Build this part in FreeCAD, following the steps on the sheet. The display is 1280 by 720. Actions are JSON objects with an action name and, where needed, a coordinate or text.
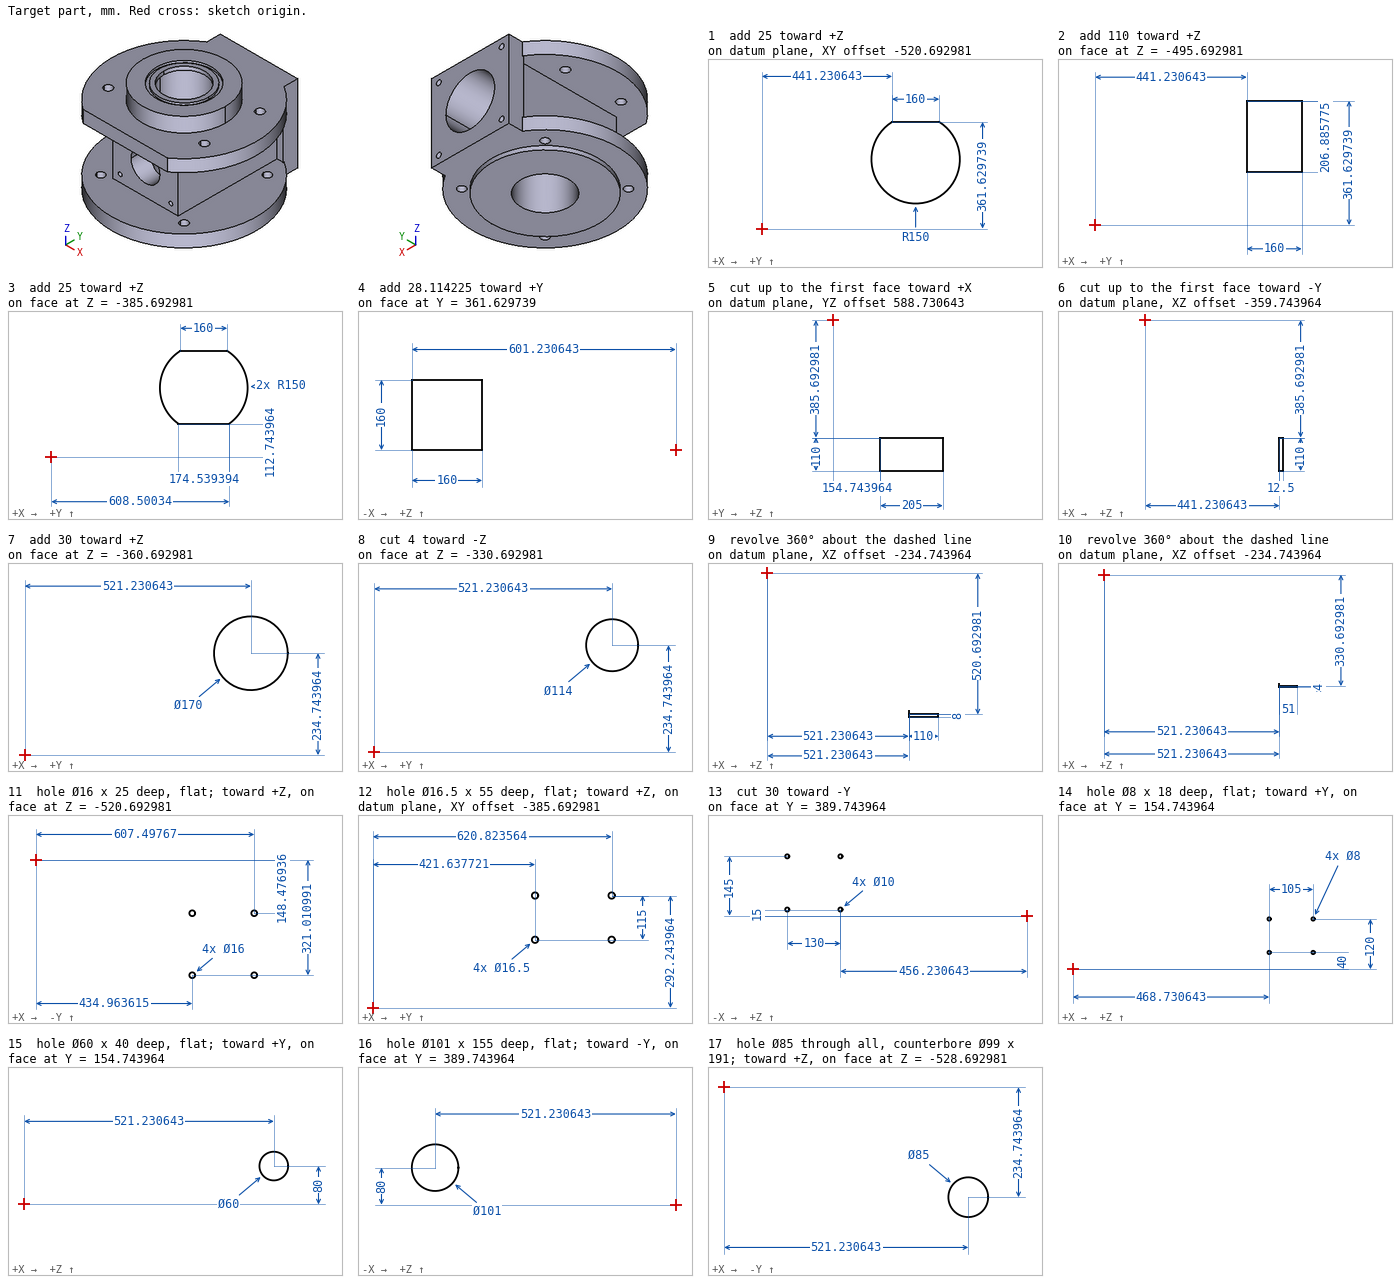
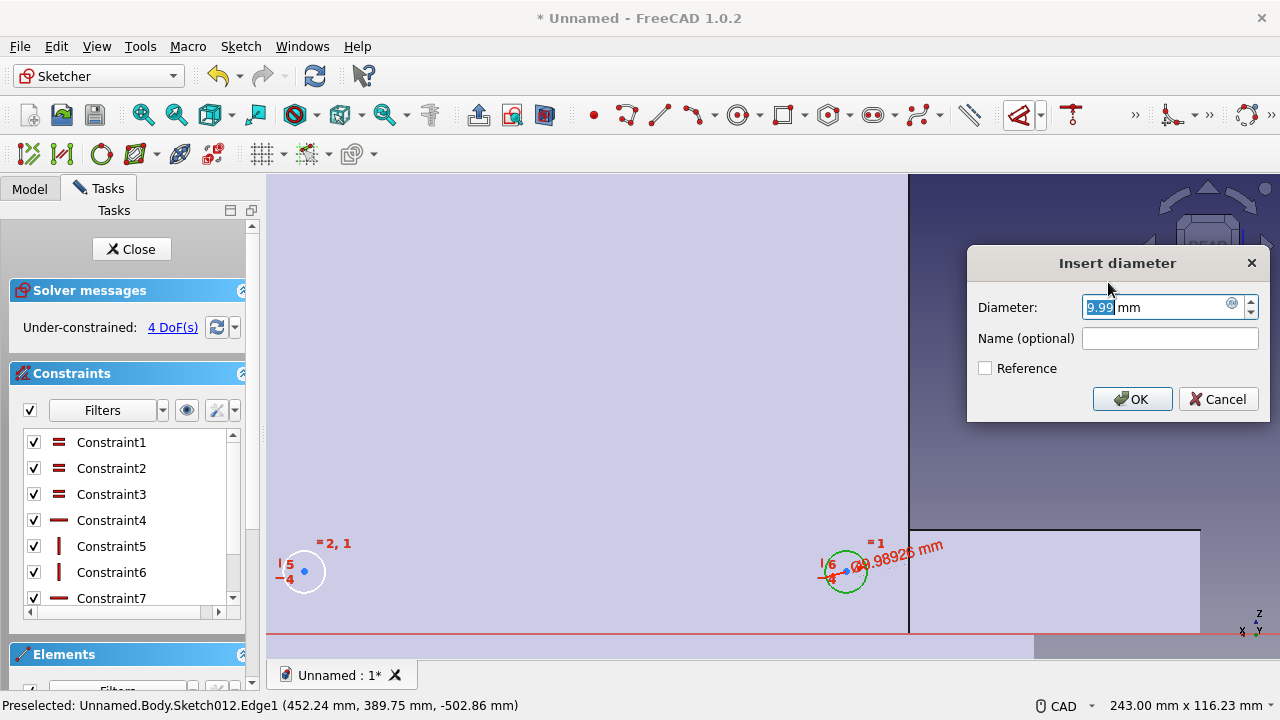
{"action": "type", "text": "10"}
{"action": "key", "text": "Return"}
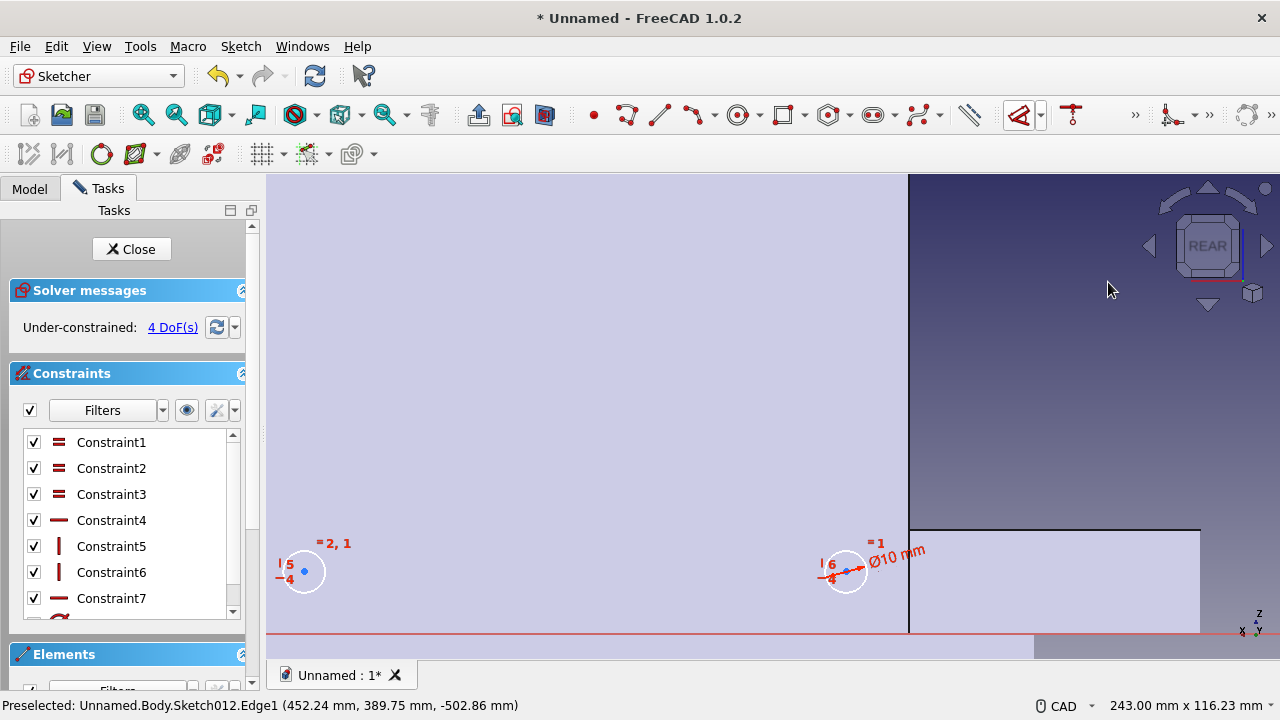
{"action": "left_click", "coordinate": [846, 572]}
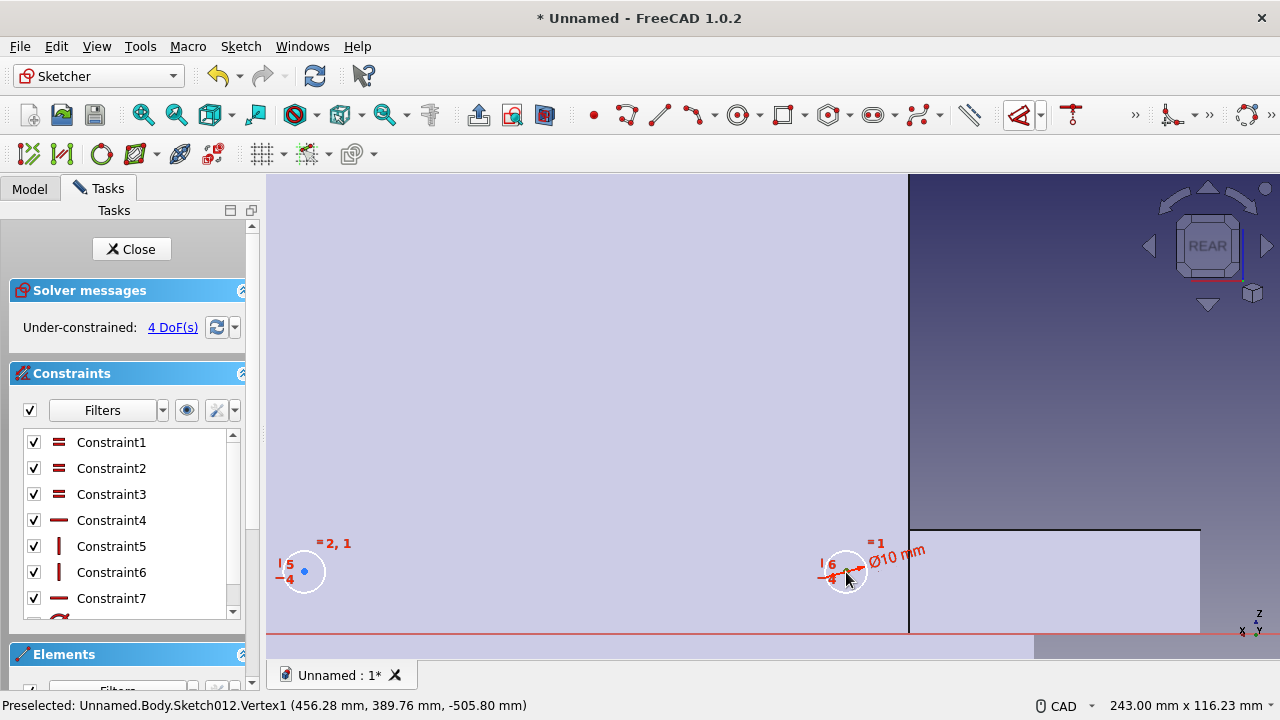
{"action": "left_click", "coordinate": [1040, 116]}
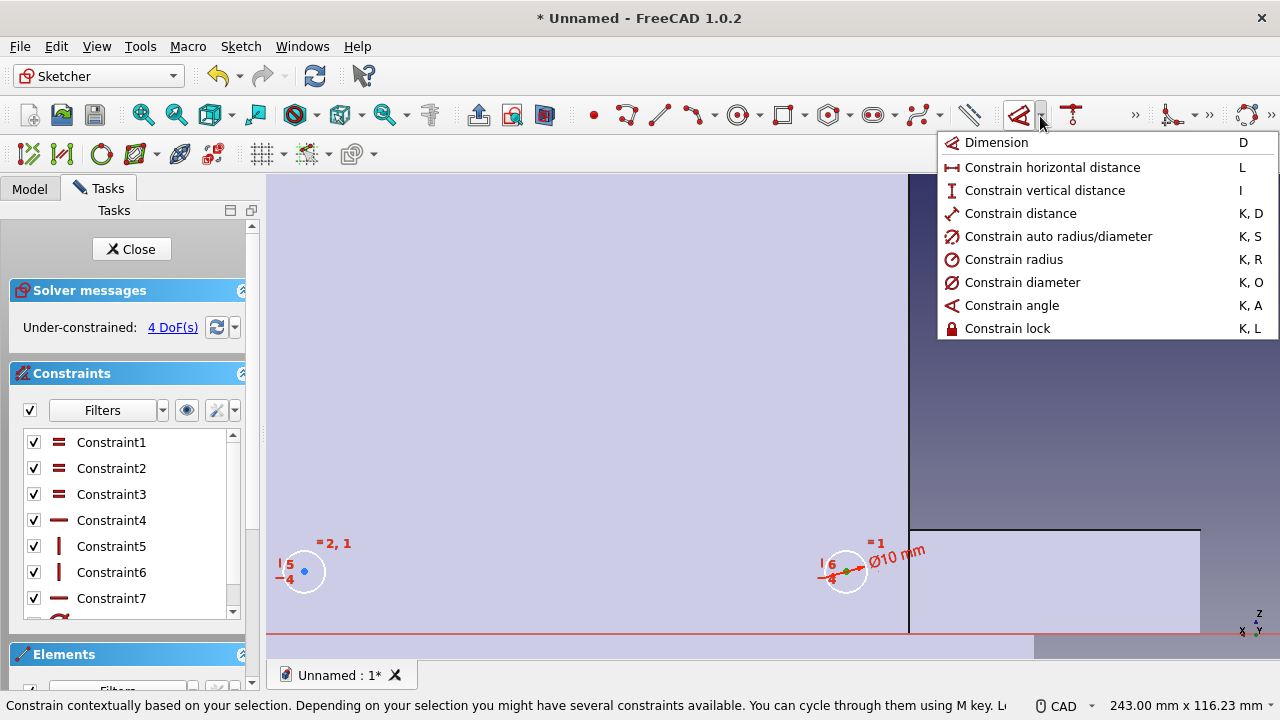
{"action": "left_click", "coordinate": [1108, 190]}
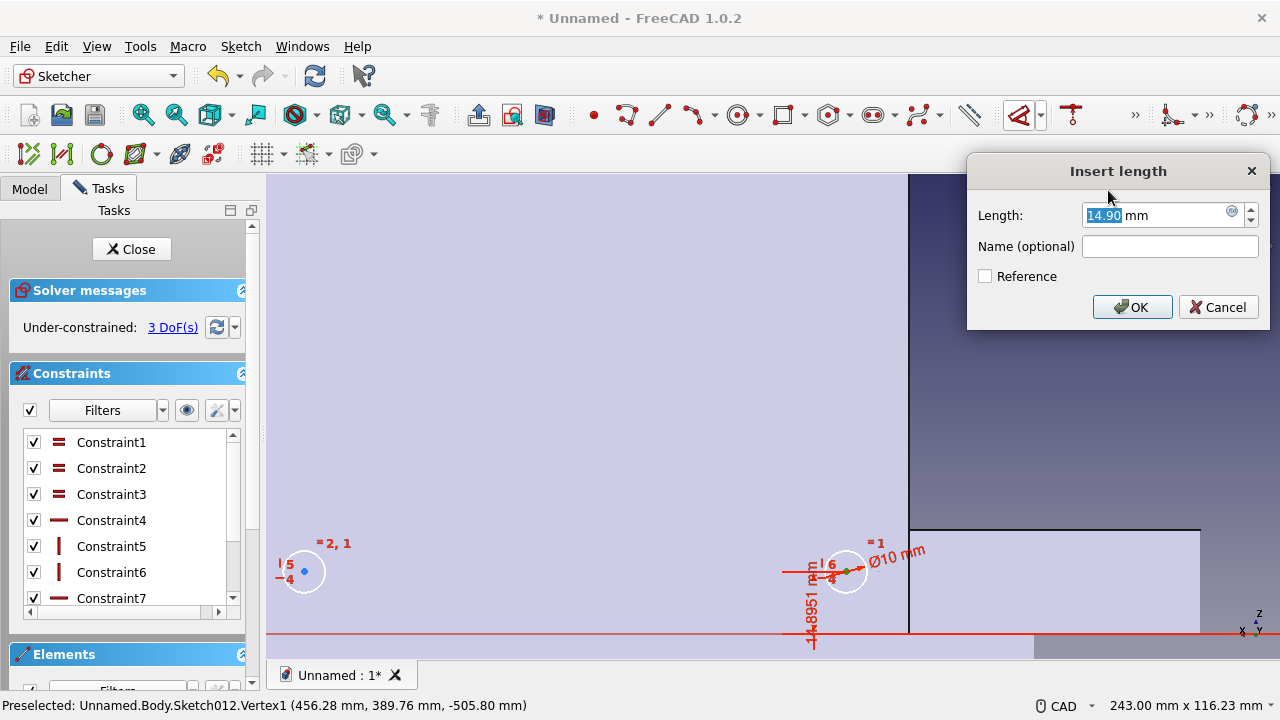
{"action": "type", "text": "15"}
{"action": "key", "text": "Return"}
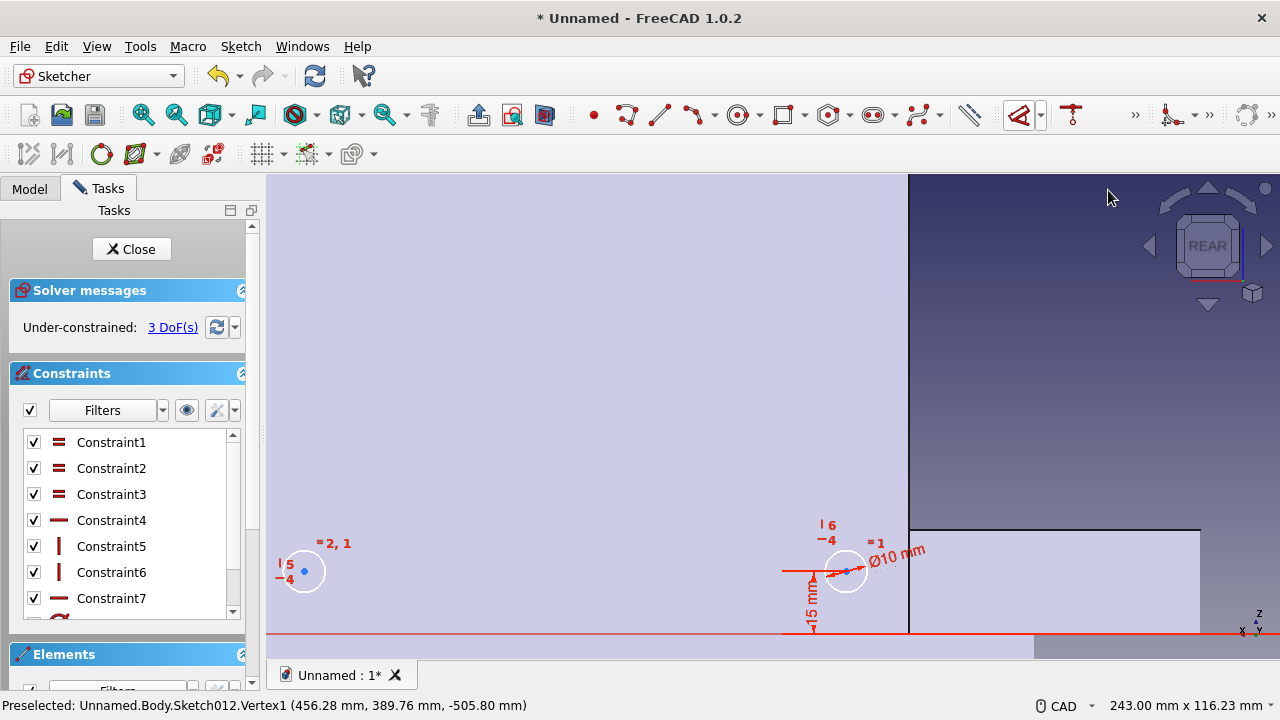
{"action": "scroll", "coordinate": [862, 558], "scroll_direction": "down", "scroll_amount": 3}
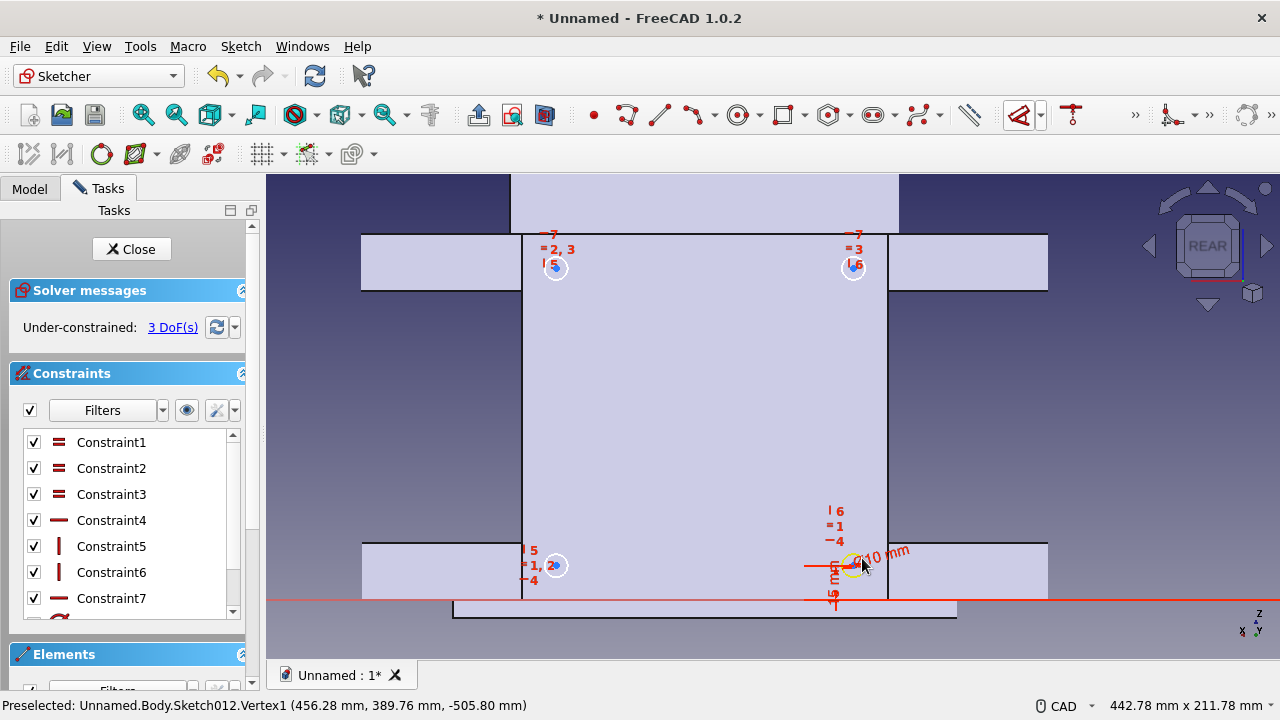
{"action": "left_click", "coordinate": [556, 268]}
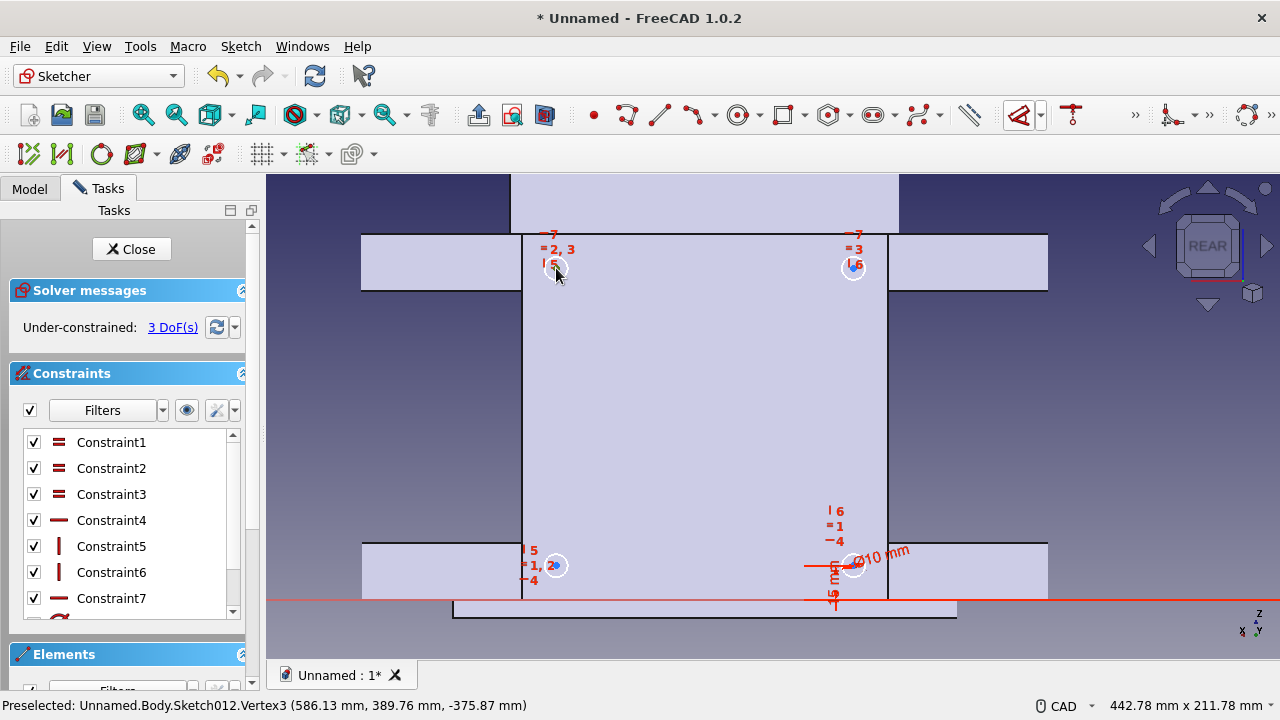
{"action": "left_click", "coordinate": [1040, 116]}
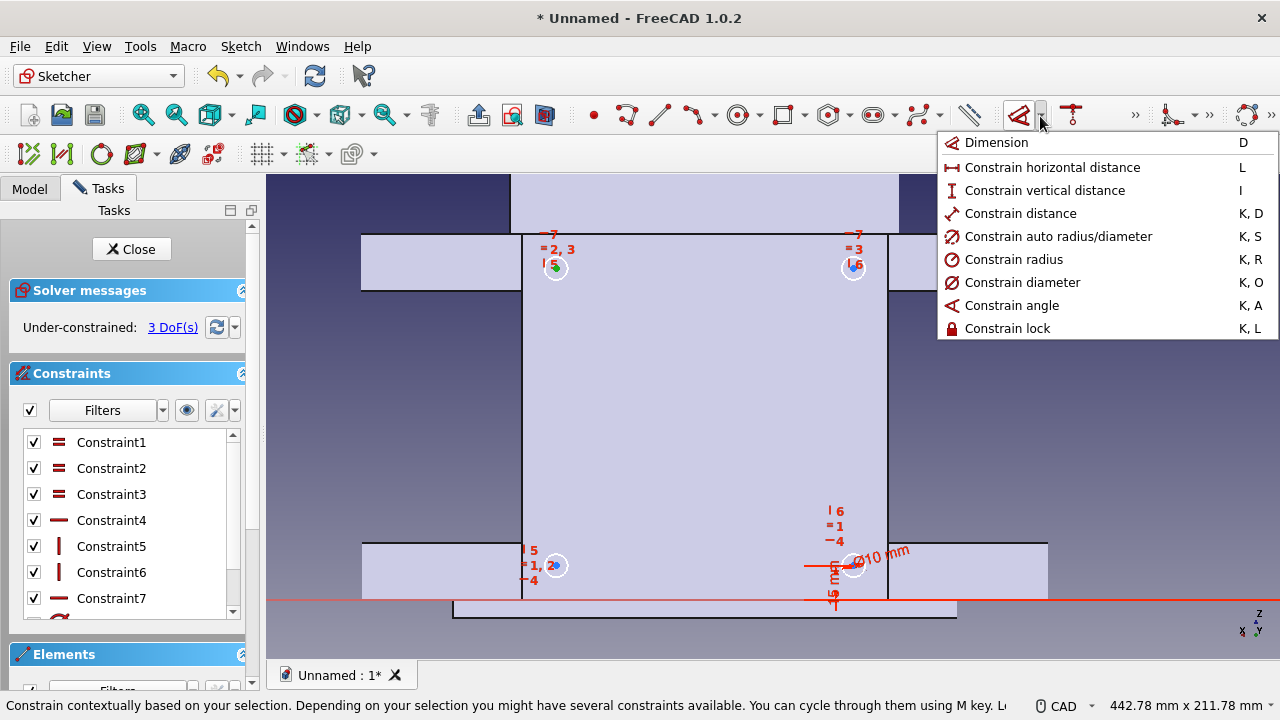
{"action": "left_click", "coordinate": [1108, 190]}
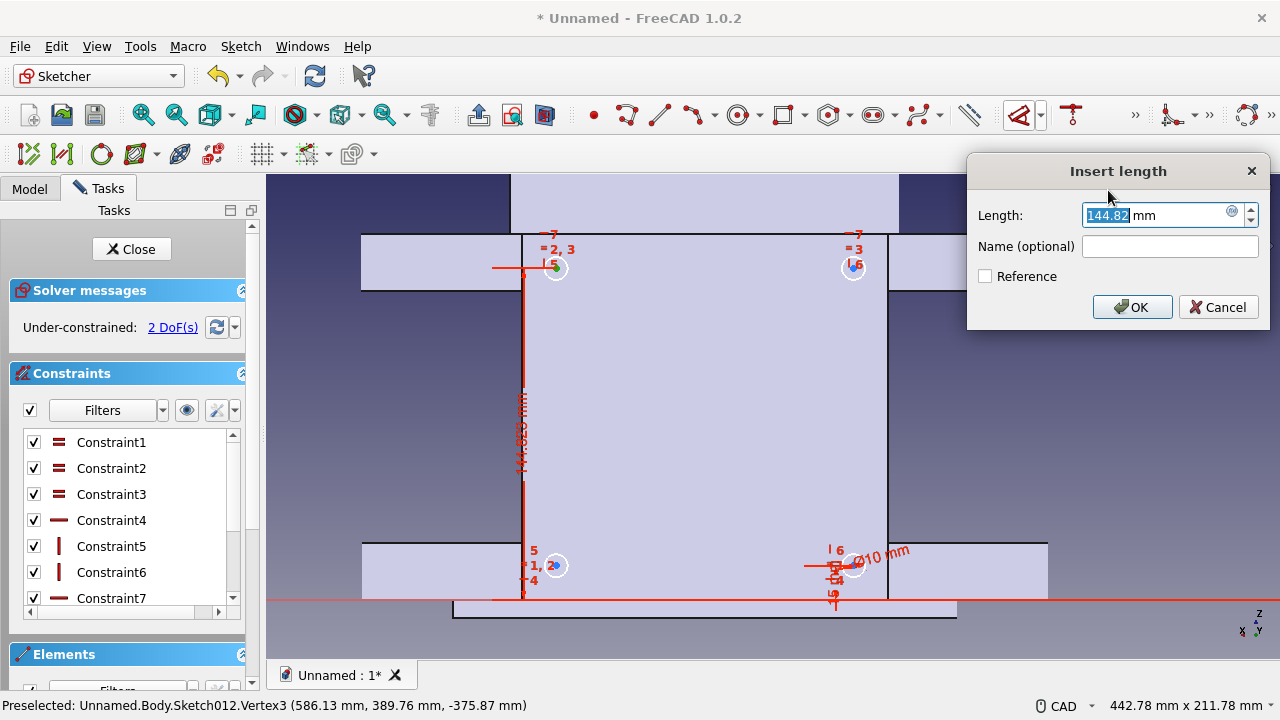
{"action": "type", "text": "145"}
{"action": "key", "text": "Return"}